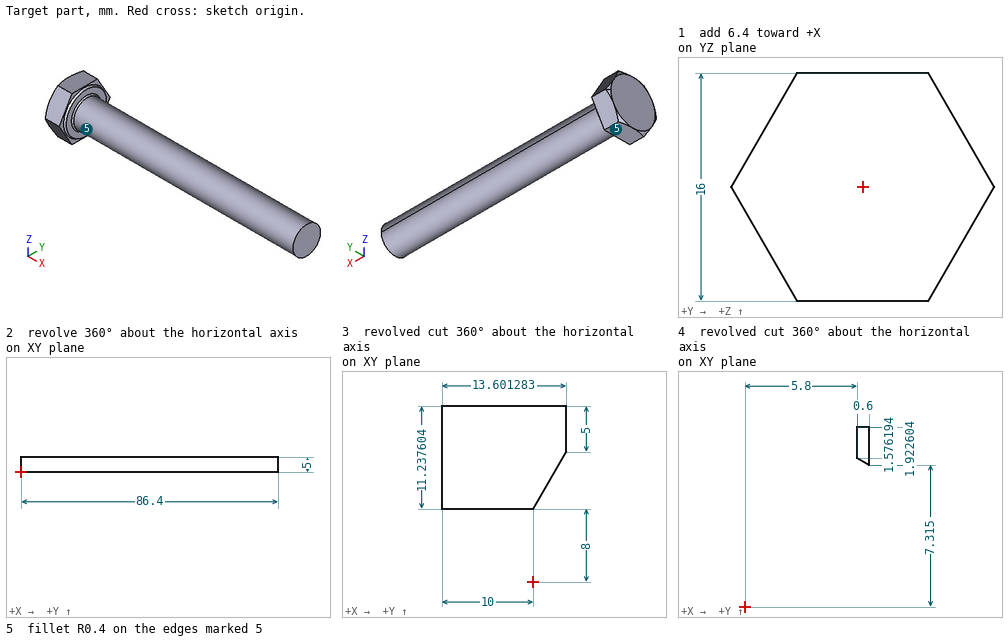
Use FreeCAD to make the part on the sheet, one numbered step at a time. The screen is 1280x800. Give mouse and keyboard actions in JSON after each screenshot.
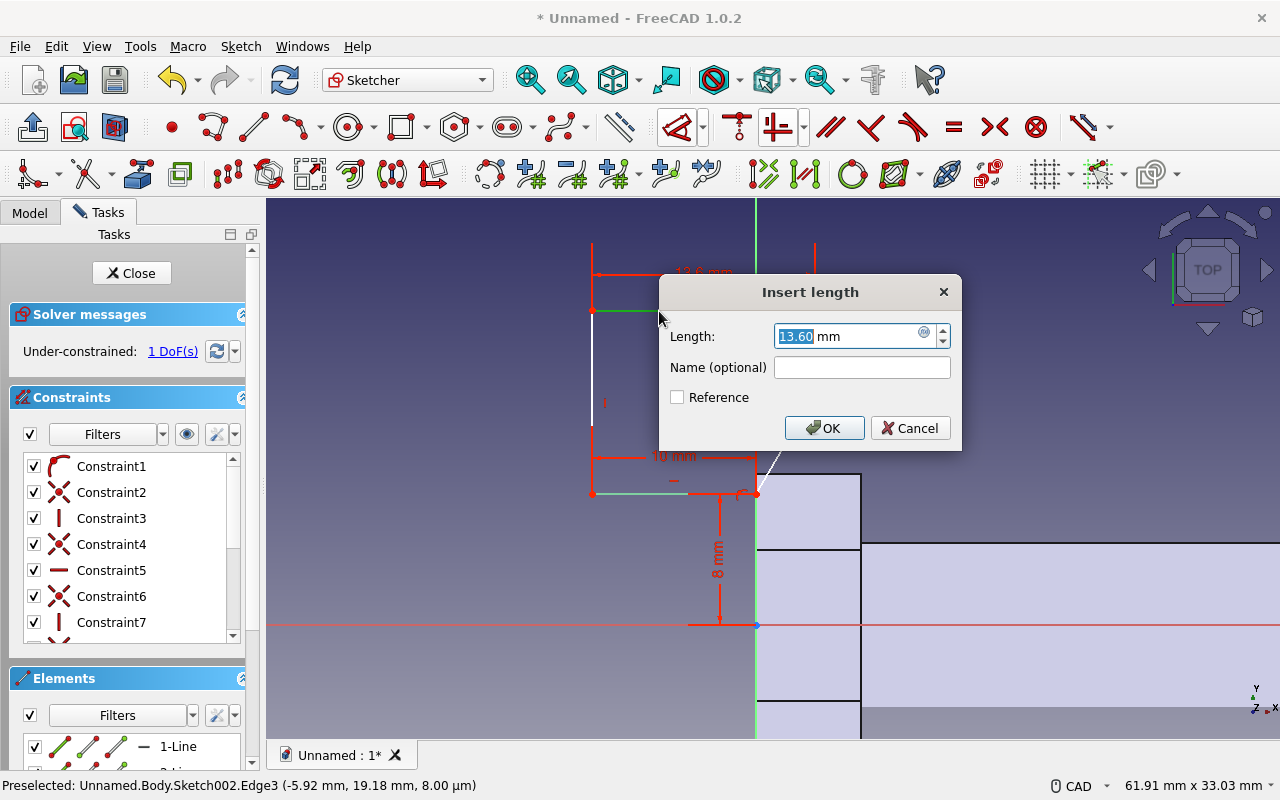
{"action": "type", "text": "13.601283"}
{"action": "key", "text": "Return"}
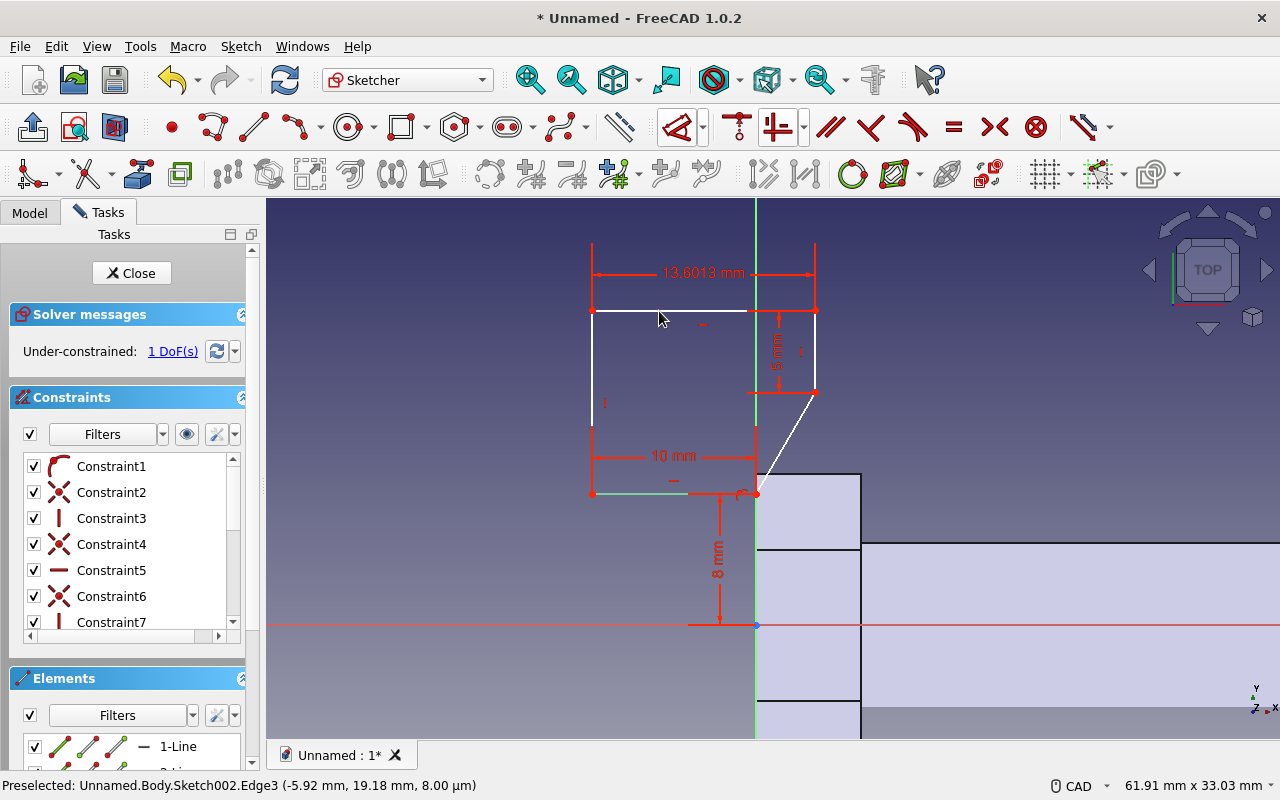
{"action": "left_click", "coordinate": [592, 366]}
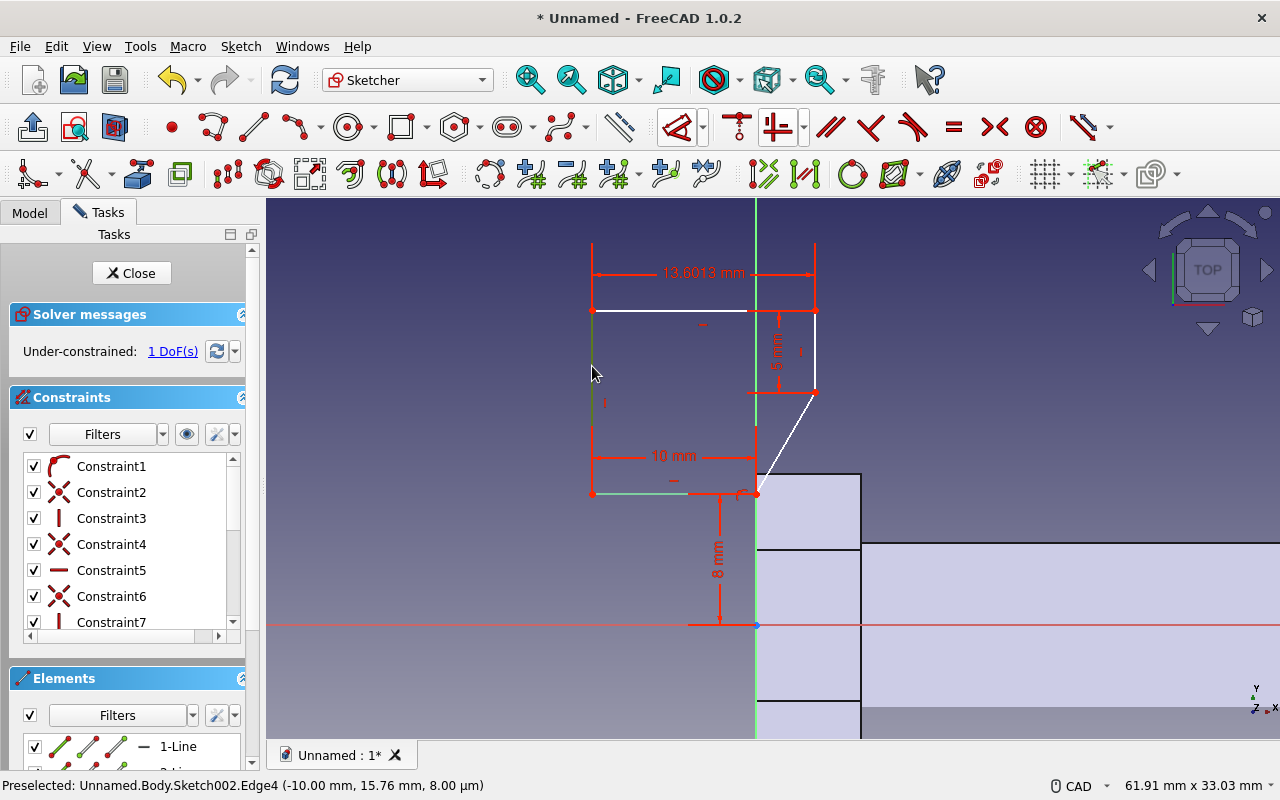
{"action": "key", "text": "i"}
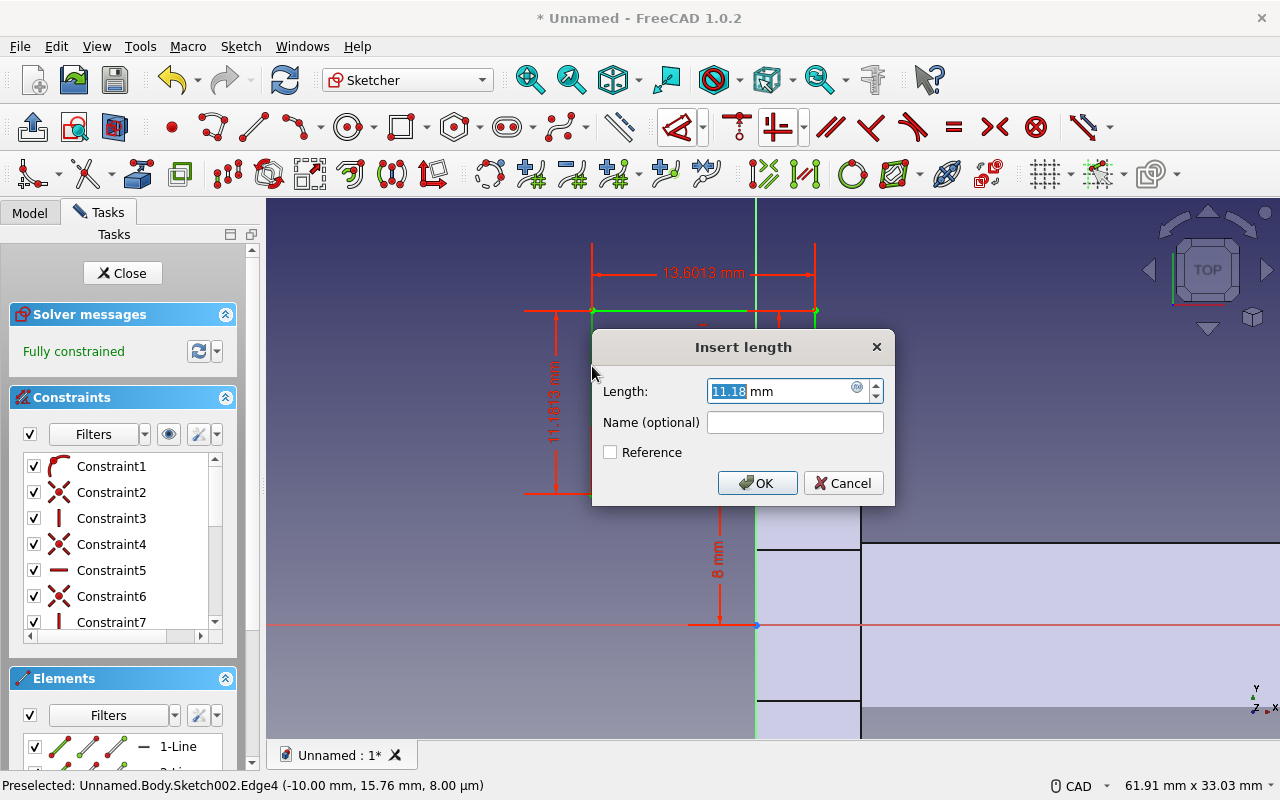
{"action": "type", "text": "11.237604"}
{"action": "key", "text": "Return"}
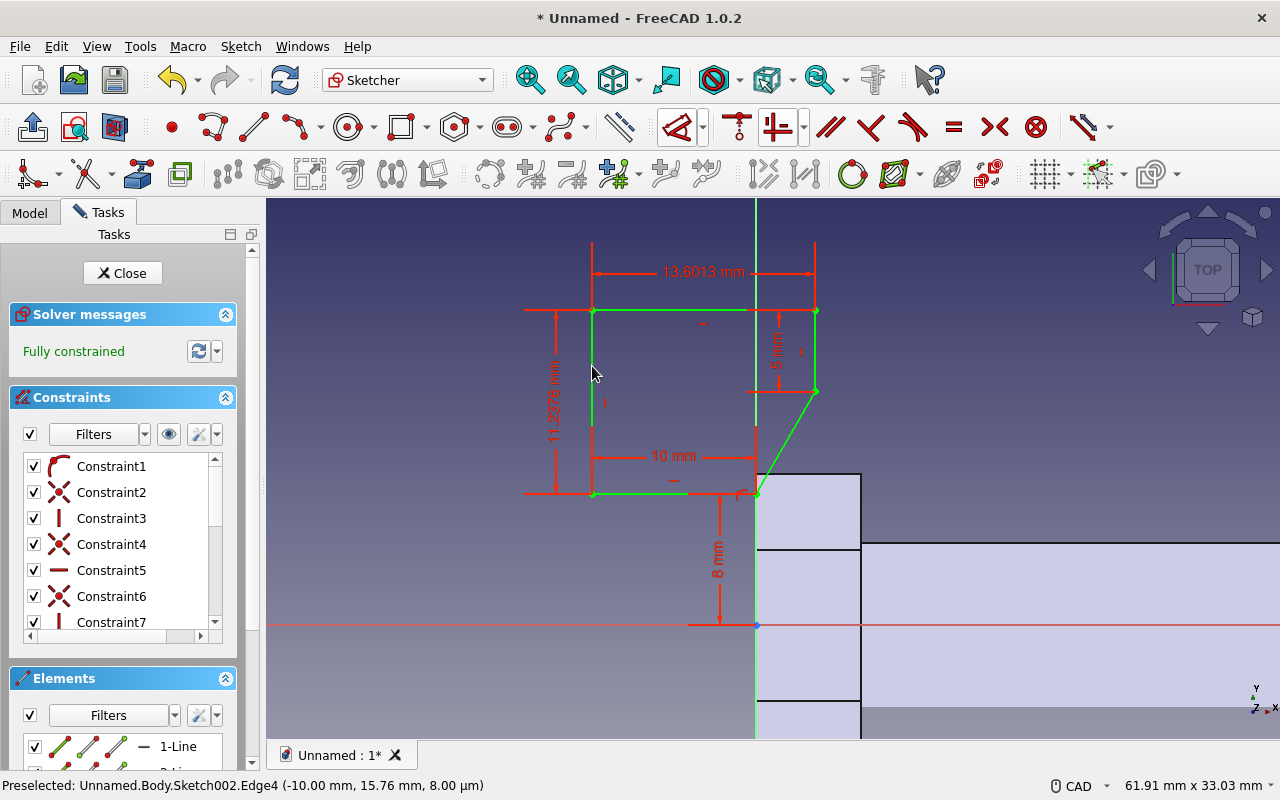
{"action": "left_click", "coordinate": [123, 273]}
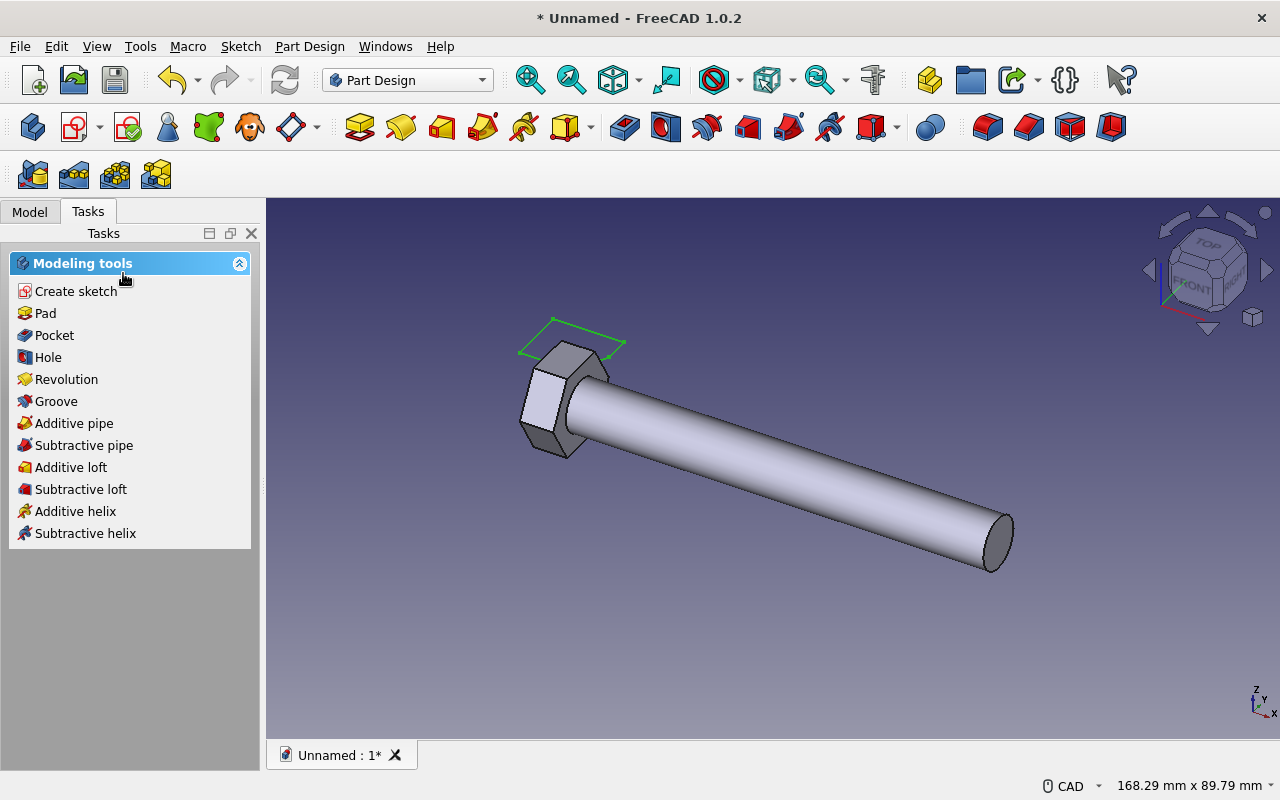
{"action": "left_click", "coordinate": [707, 128]}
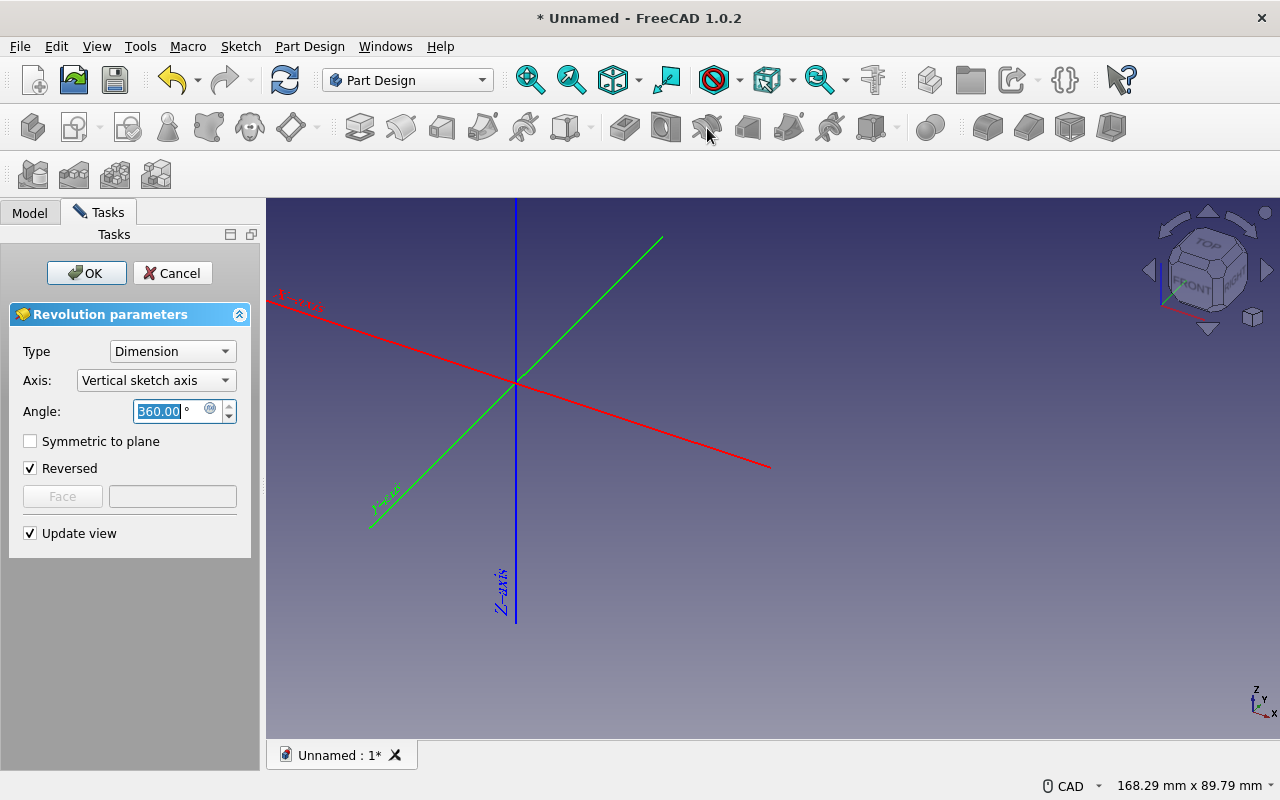
{"action": "left_click", "coordinate": [157, 380]}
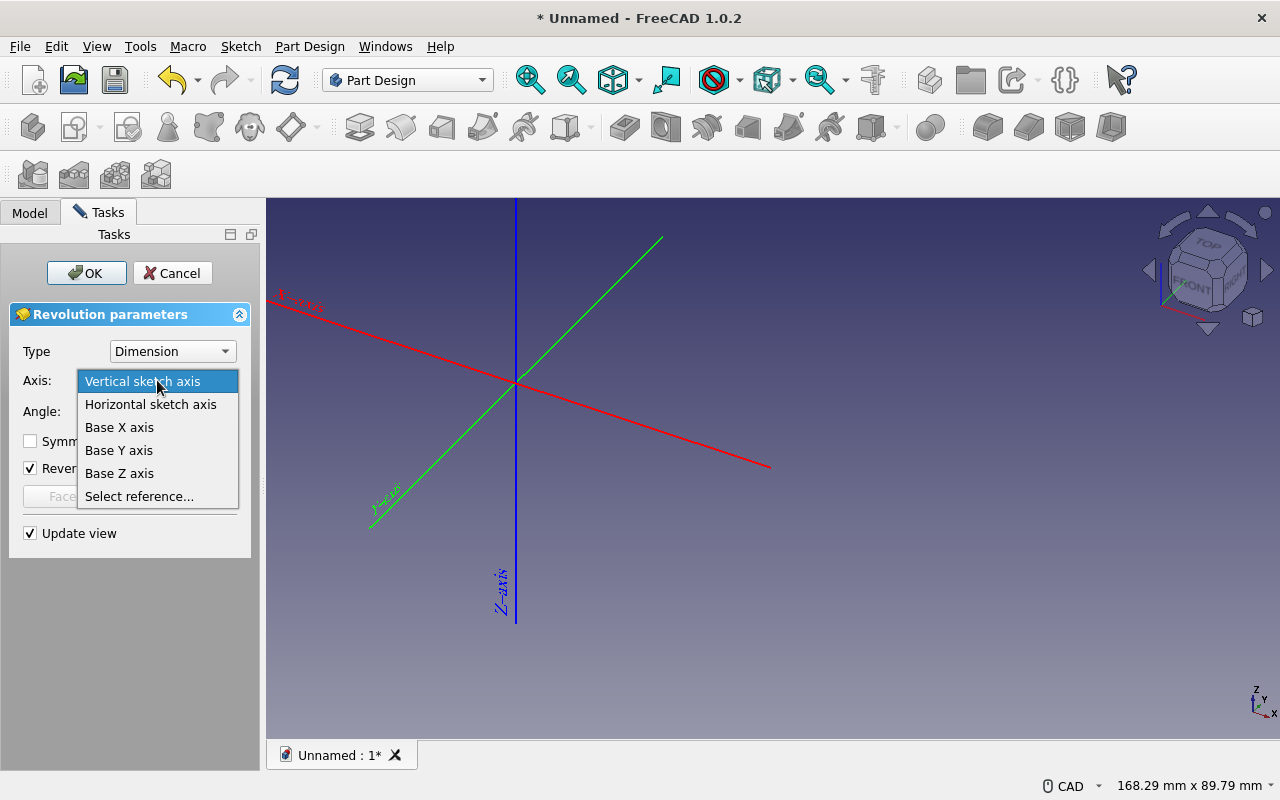
{"action": "left_click", "coordinate": [156, 404]}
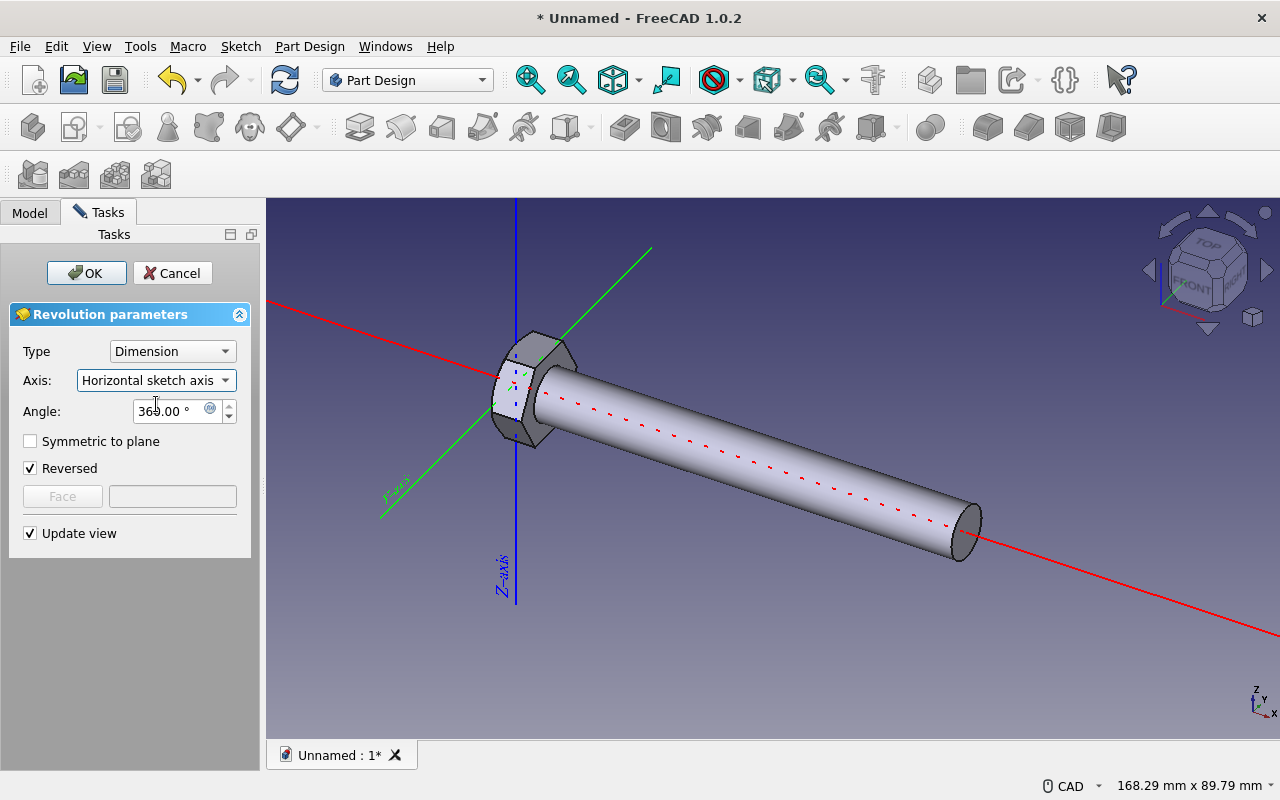
{"action": "left_click", "coordinate": [87, 273]}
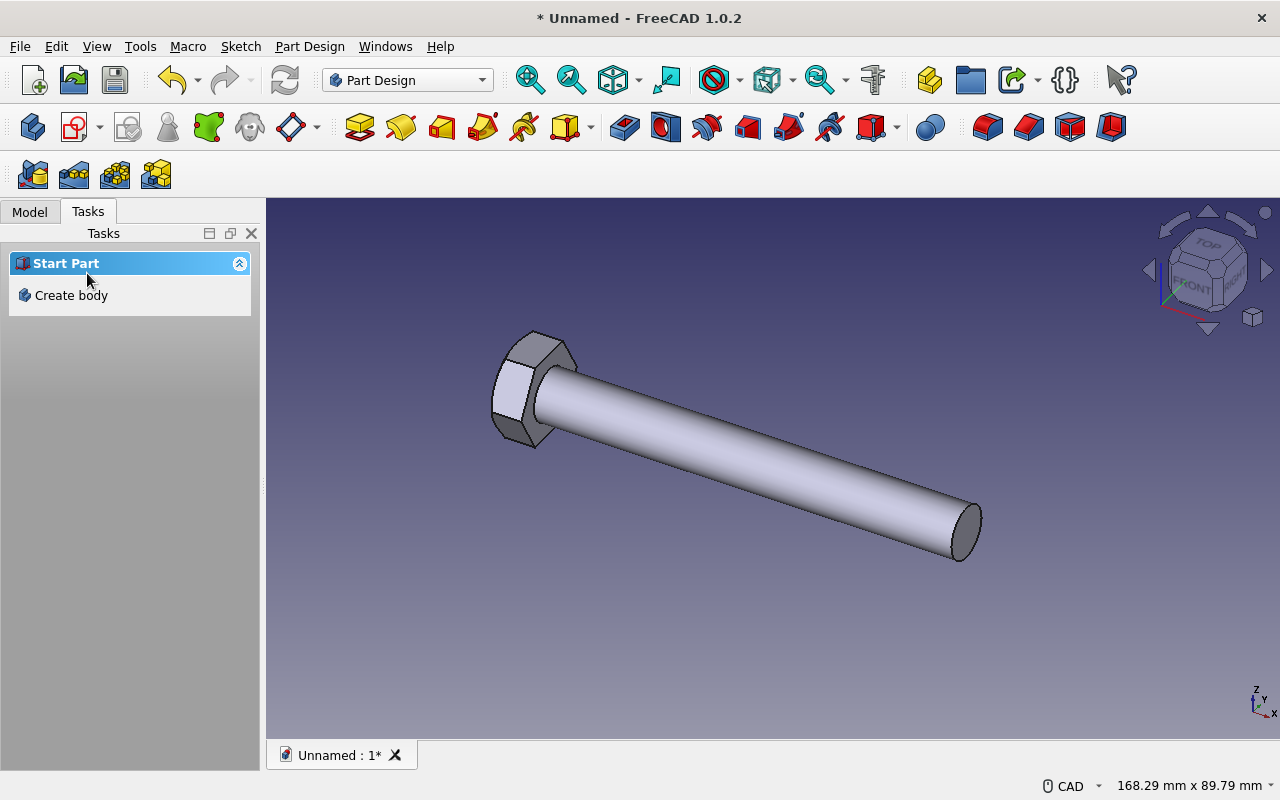
{"action": "left_click", "coordinate": [74, 128]}